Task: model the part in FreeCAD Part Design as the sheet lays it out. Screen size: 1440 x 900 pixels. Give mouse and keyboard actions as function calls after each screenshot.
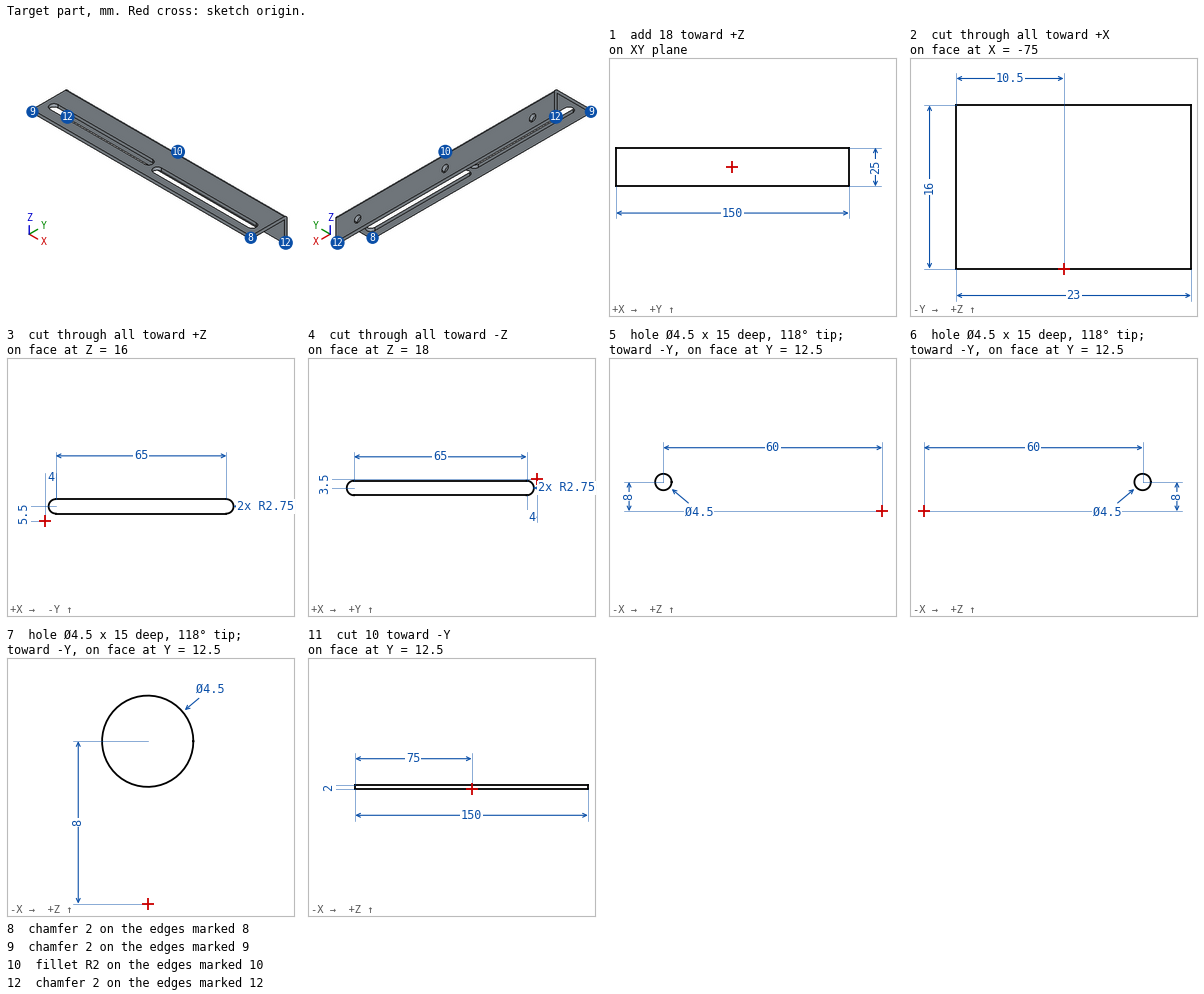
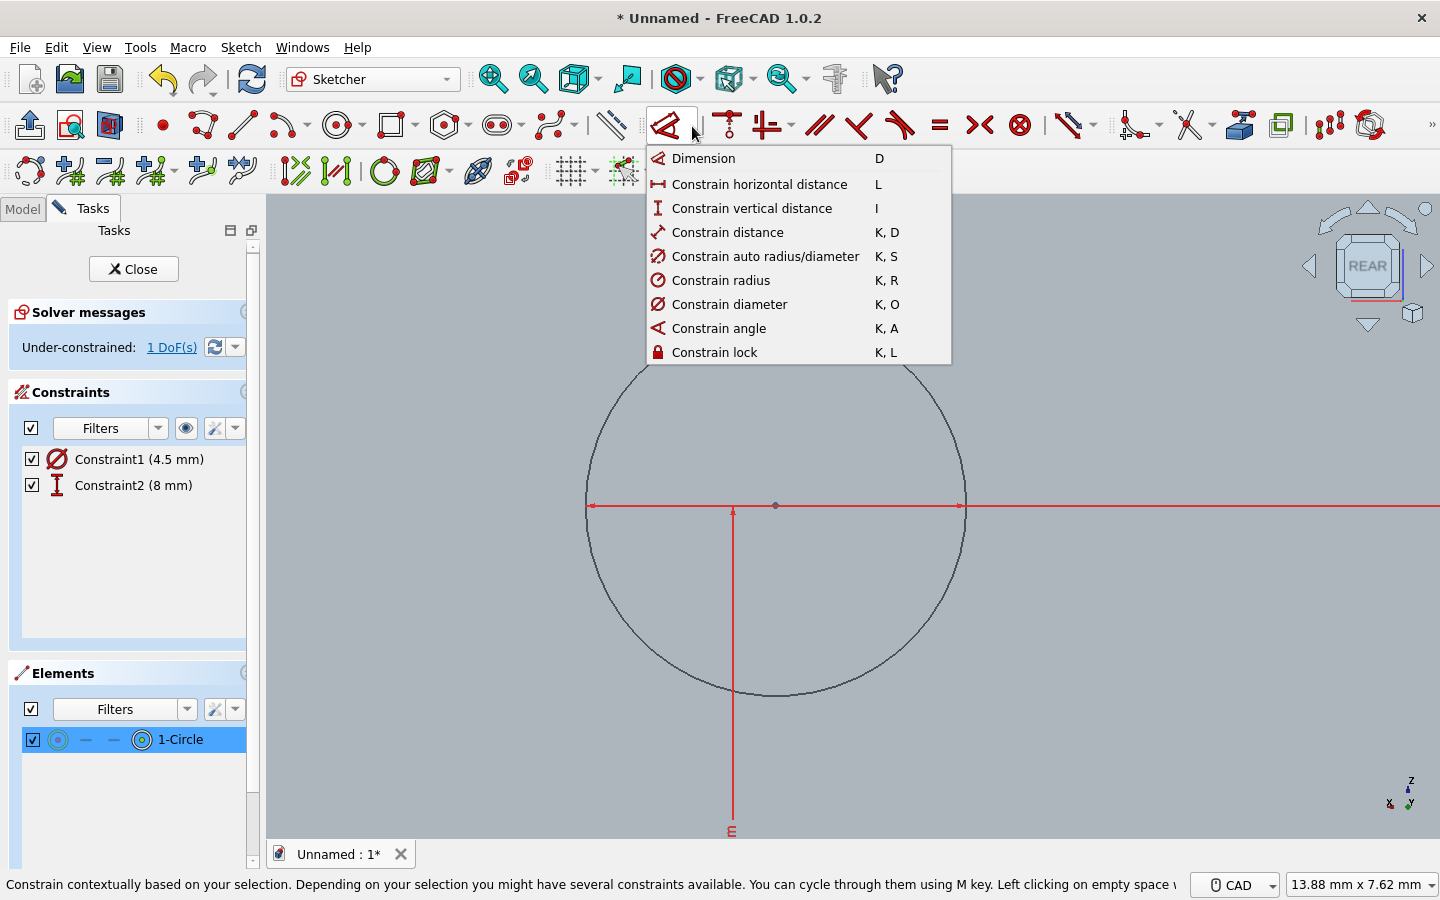
click(799, 184)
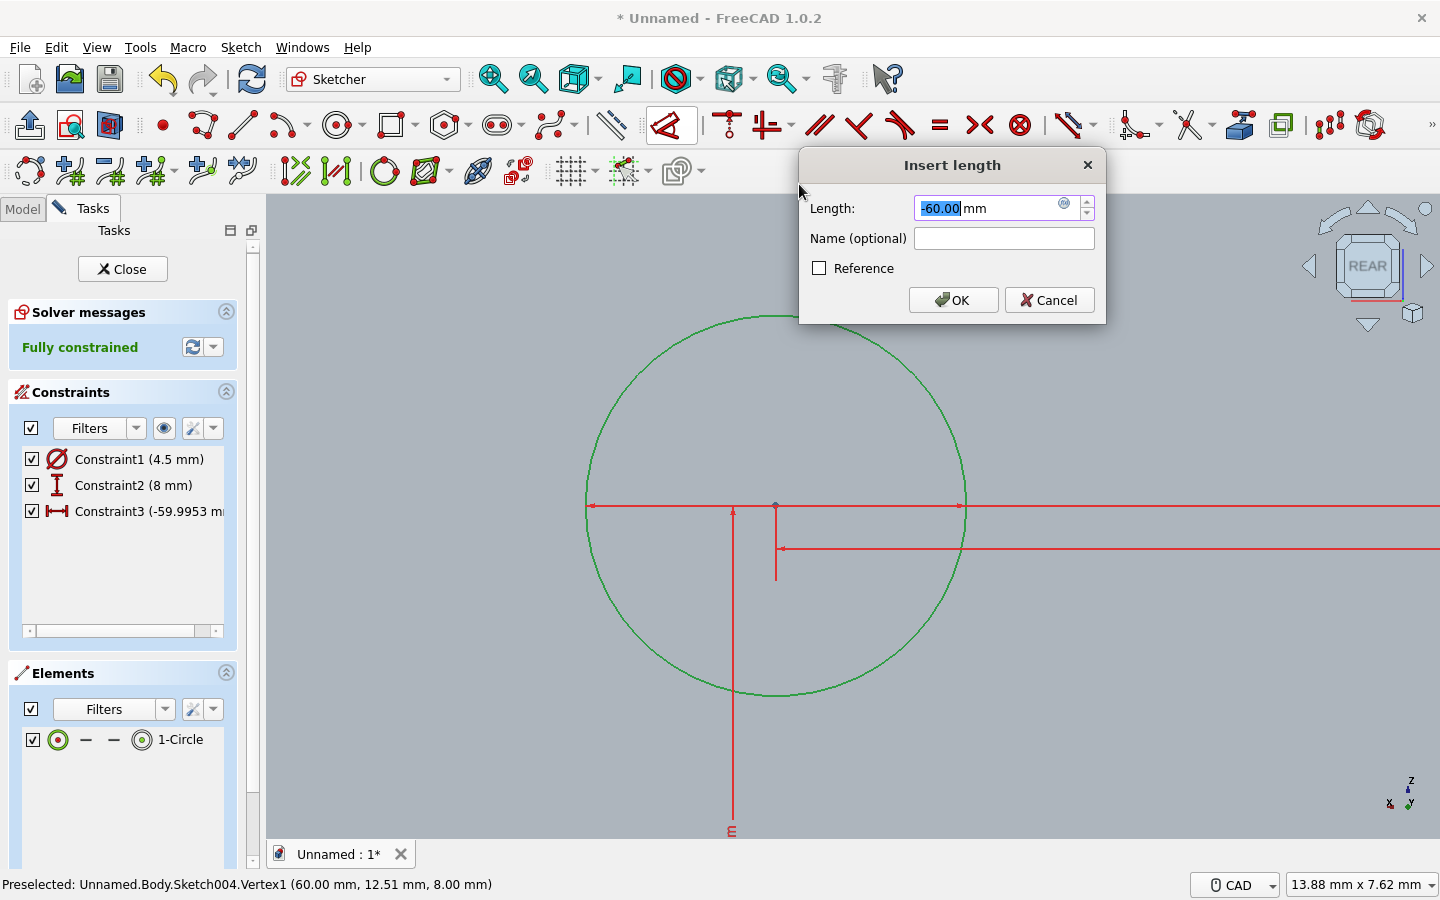
text(-60)
key(Return)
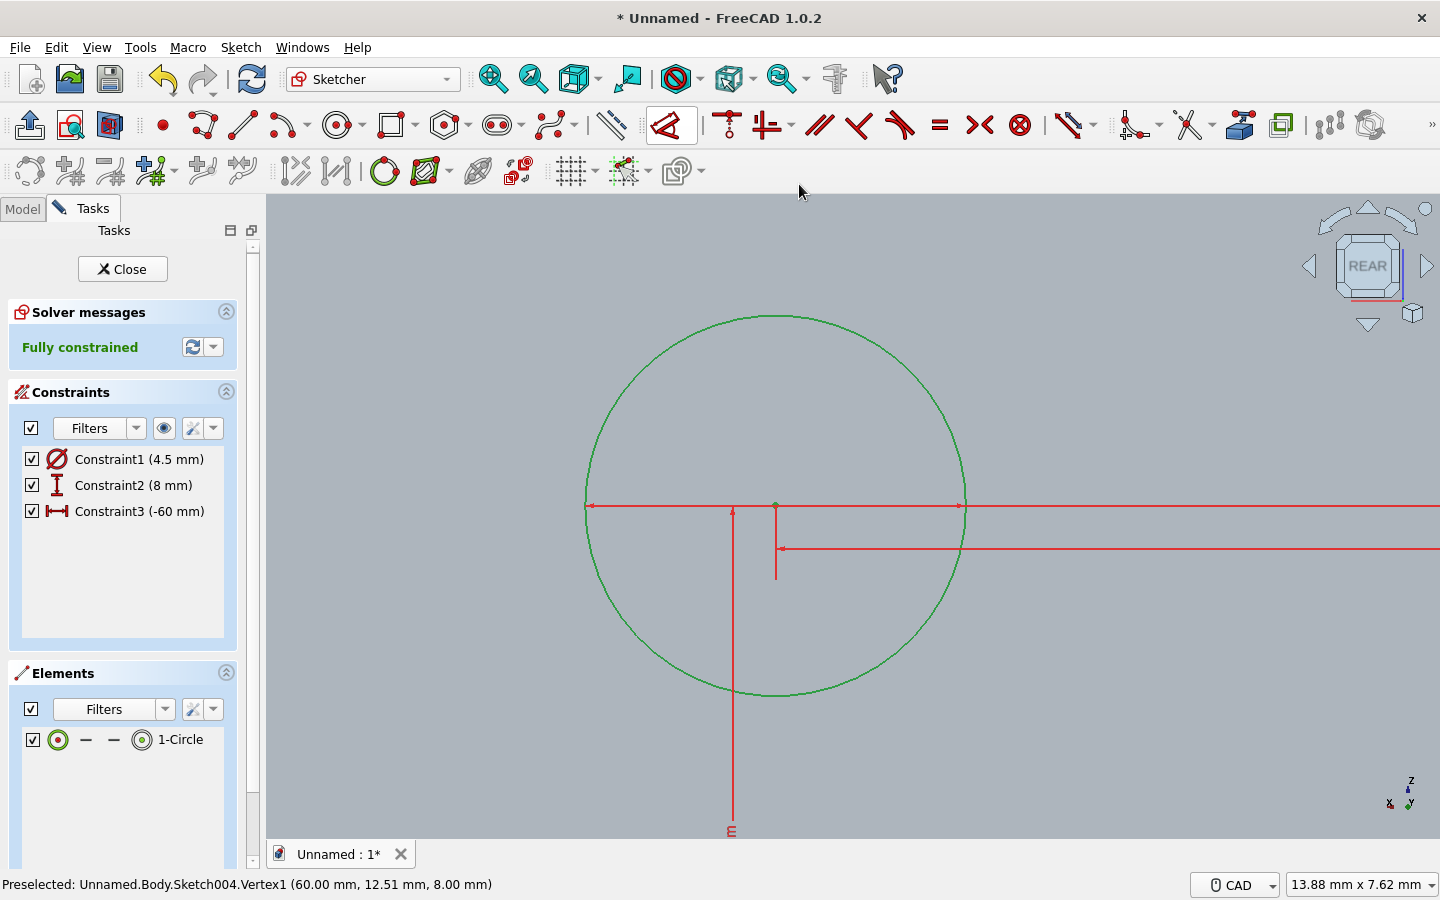
click(123, 269)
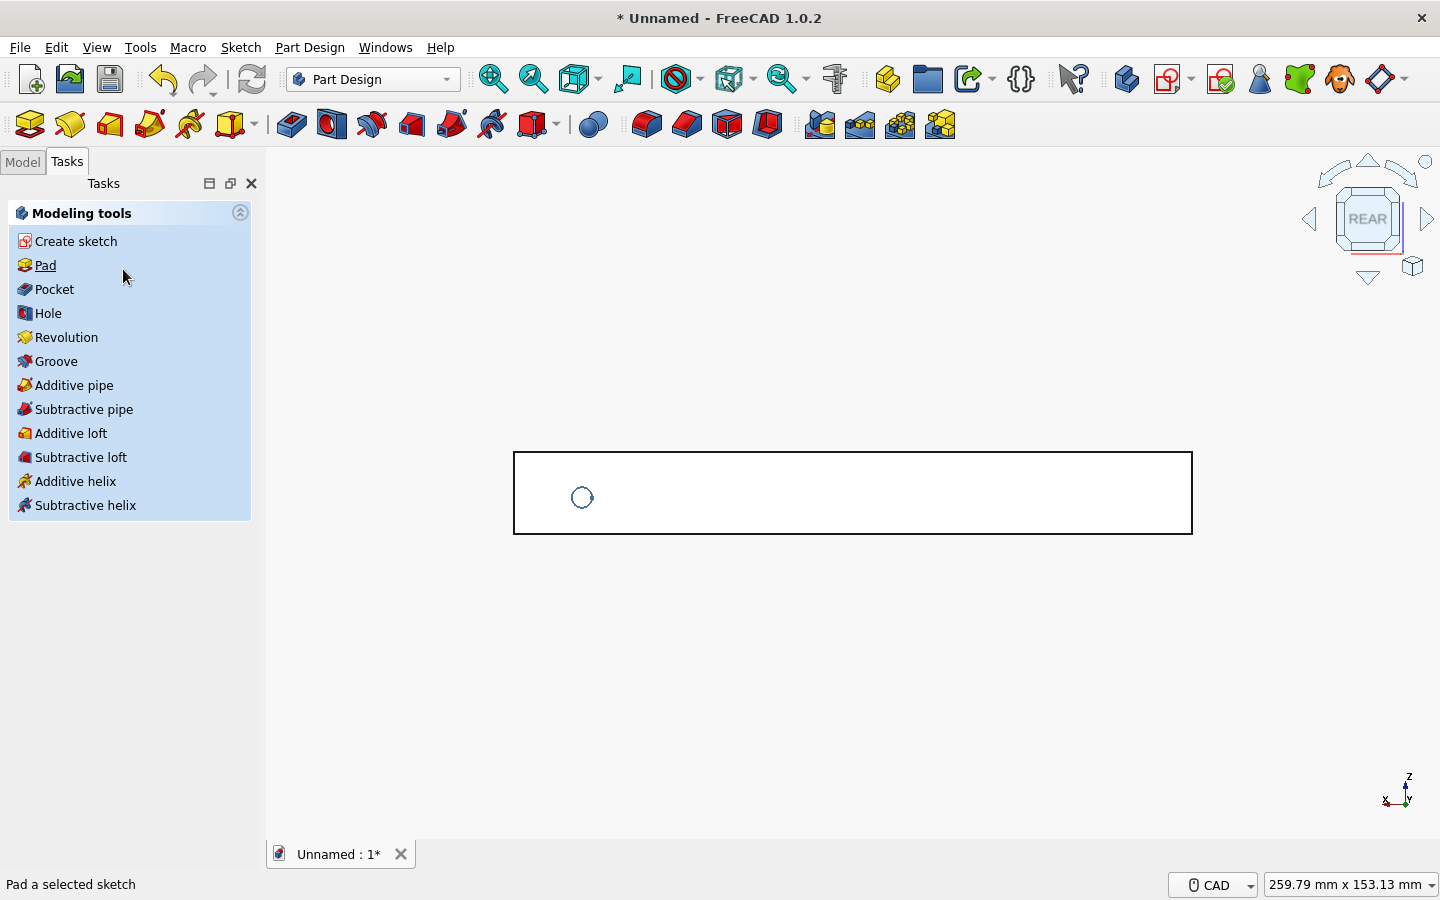
click(332, 124)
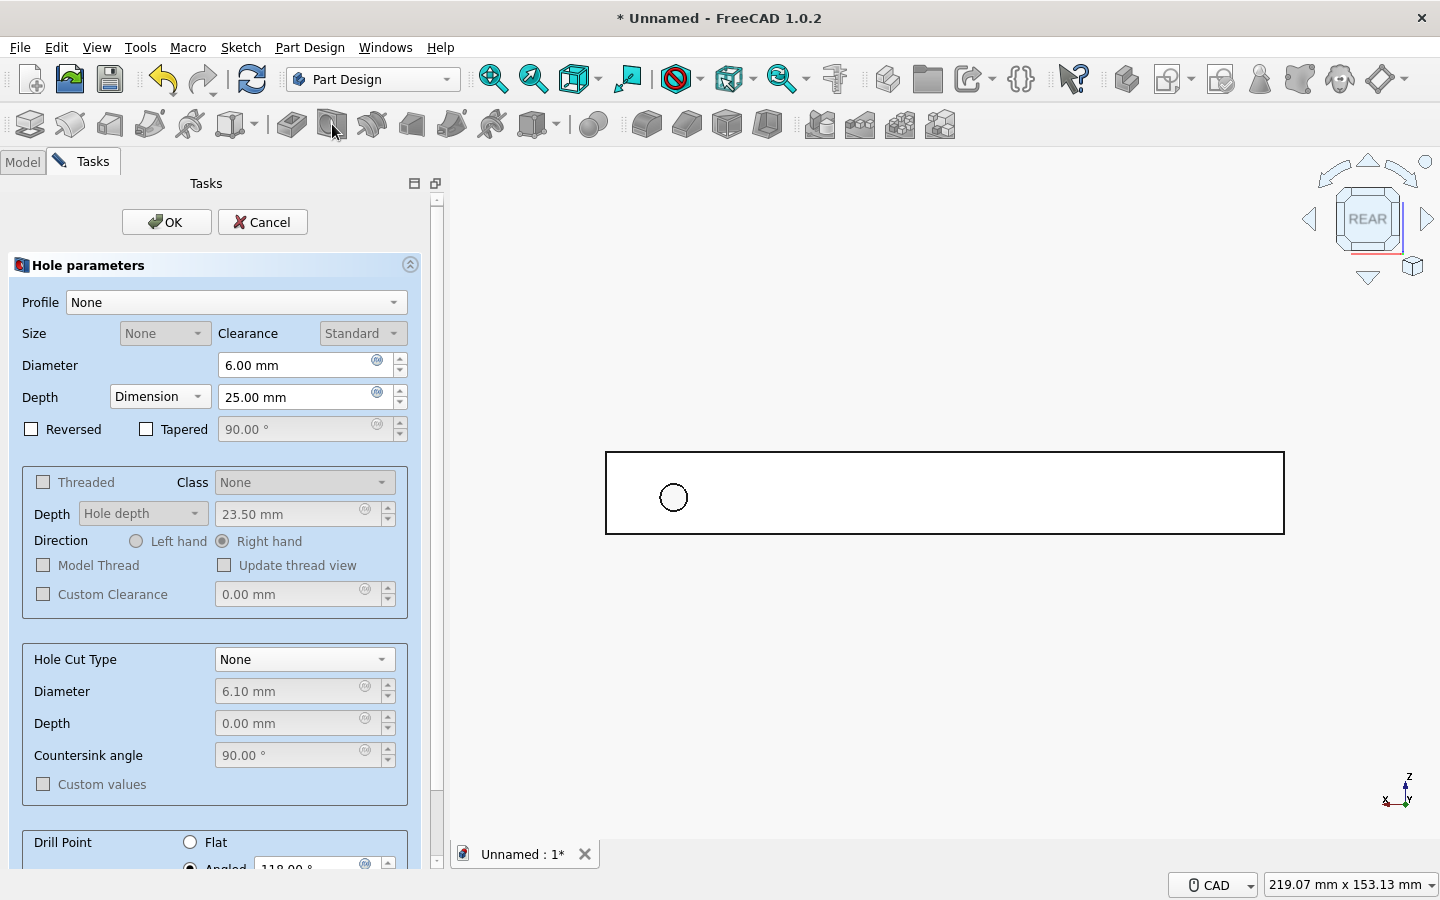
triple_click(305, 365)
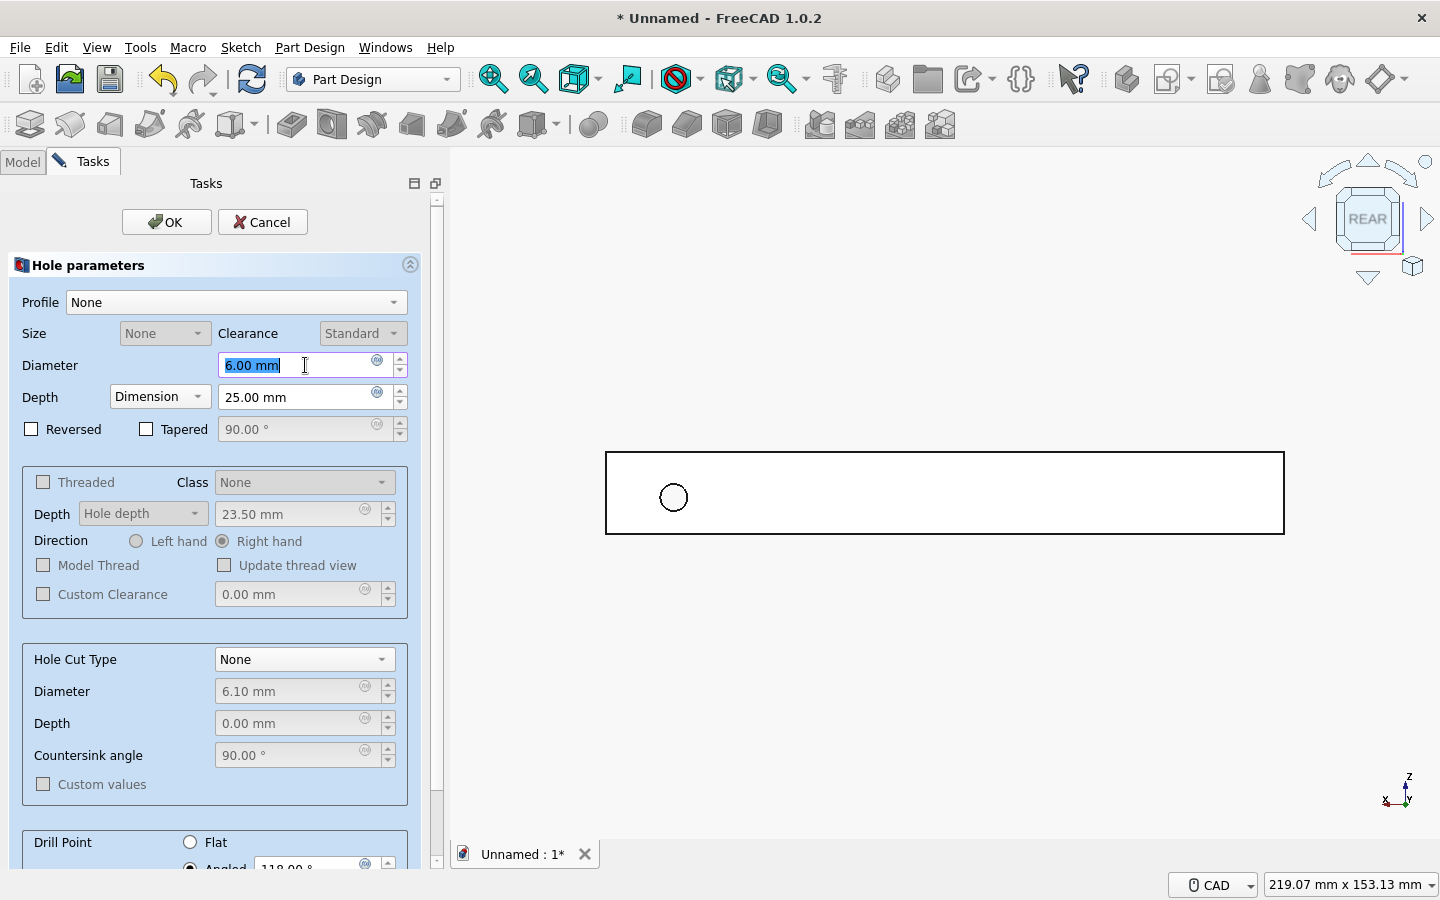
text(4.5)
key(Tab)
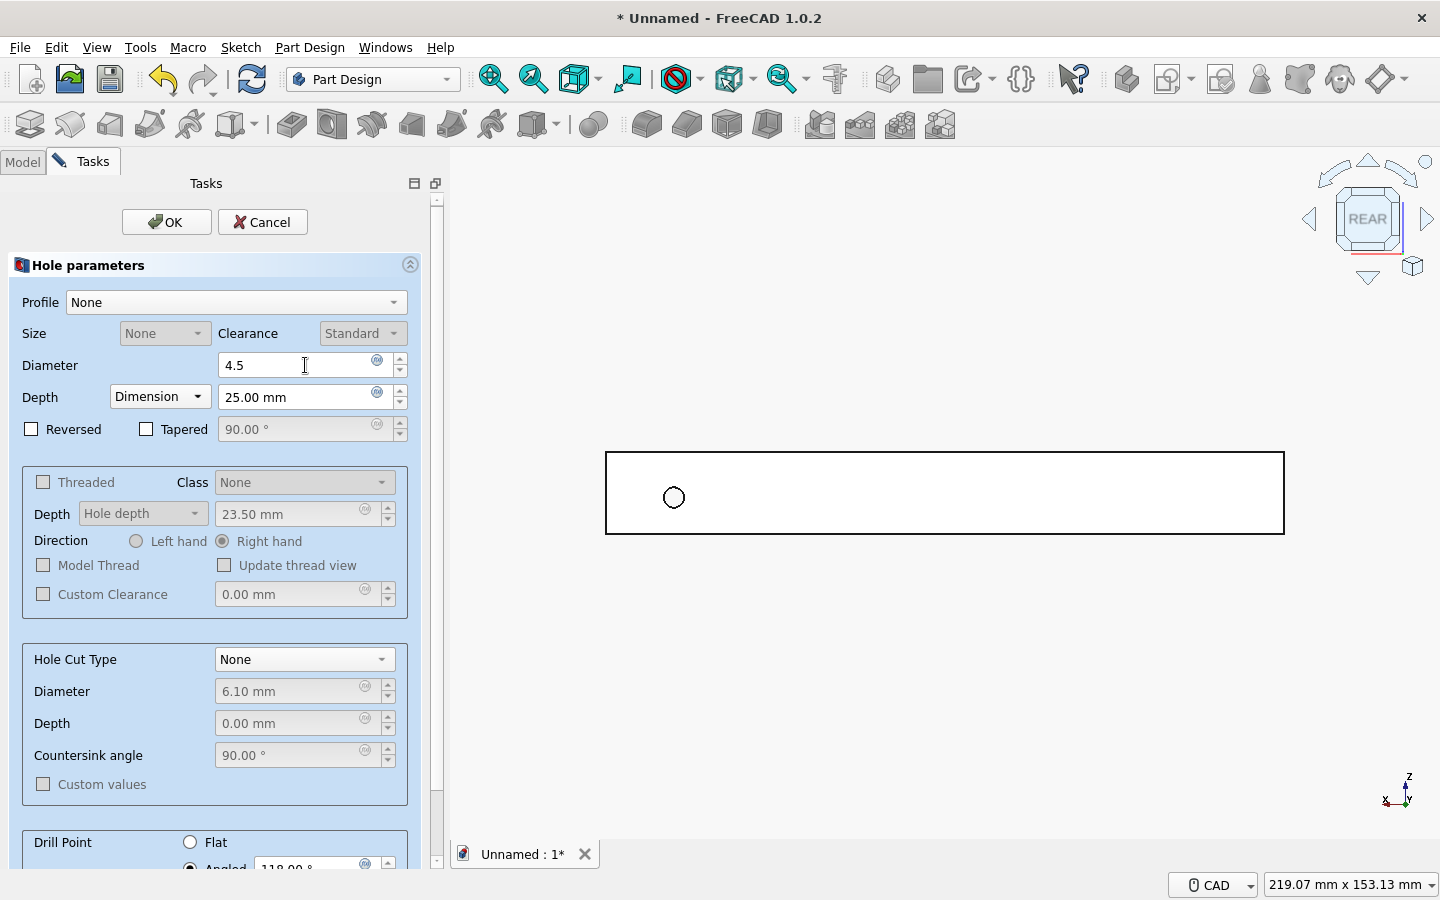
triple_click(305, 397)